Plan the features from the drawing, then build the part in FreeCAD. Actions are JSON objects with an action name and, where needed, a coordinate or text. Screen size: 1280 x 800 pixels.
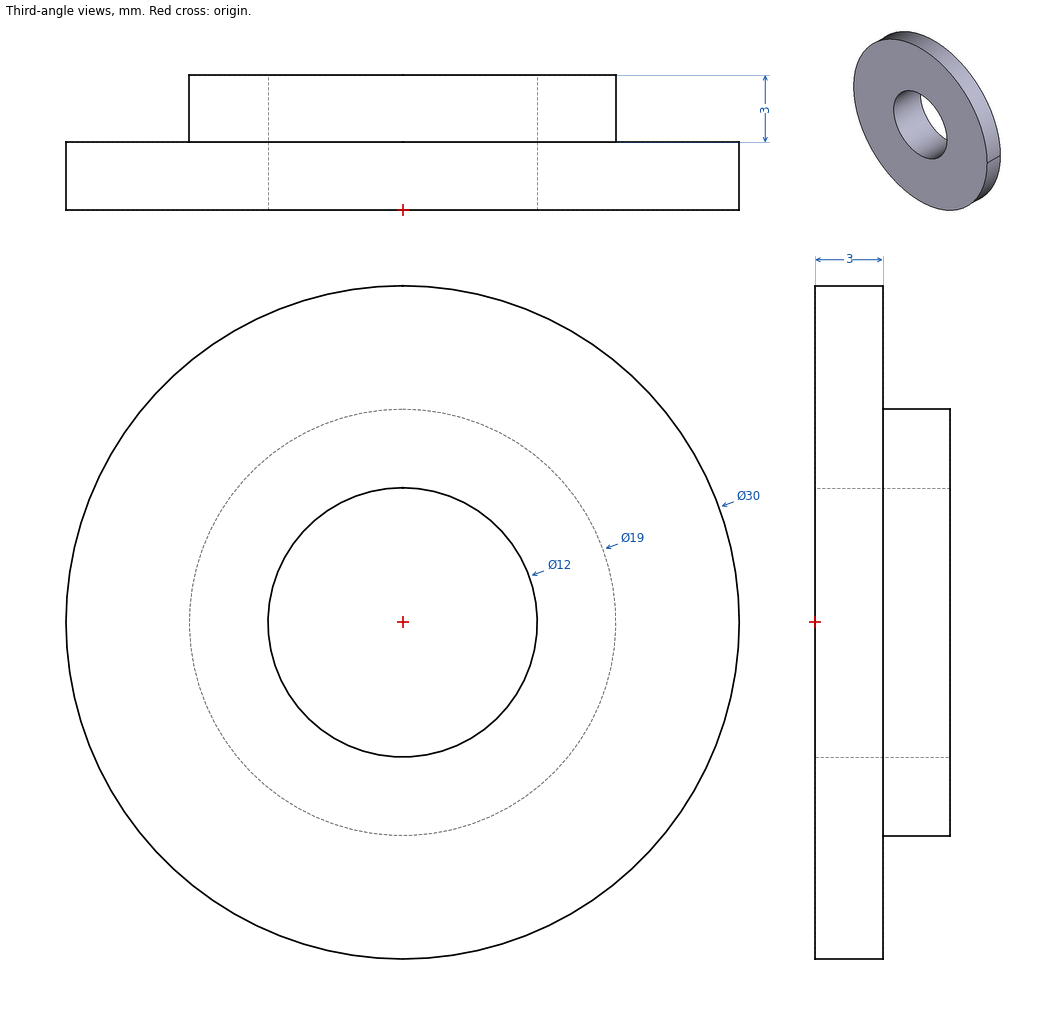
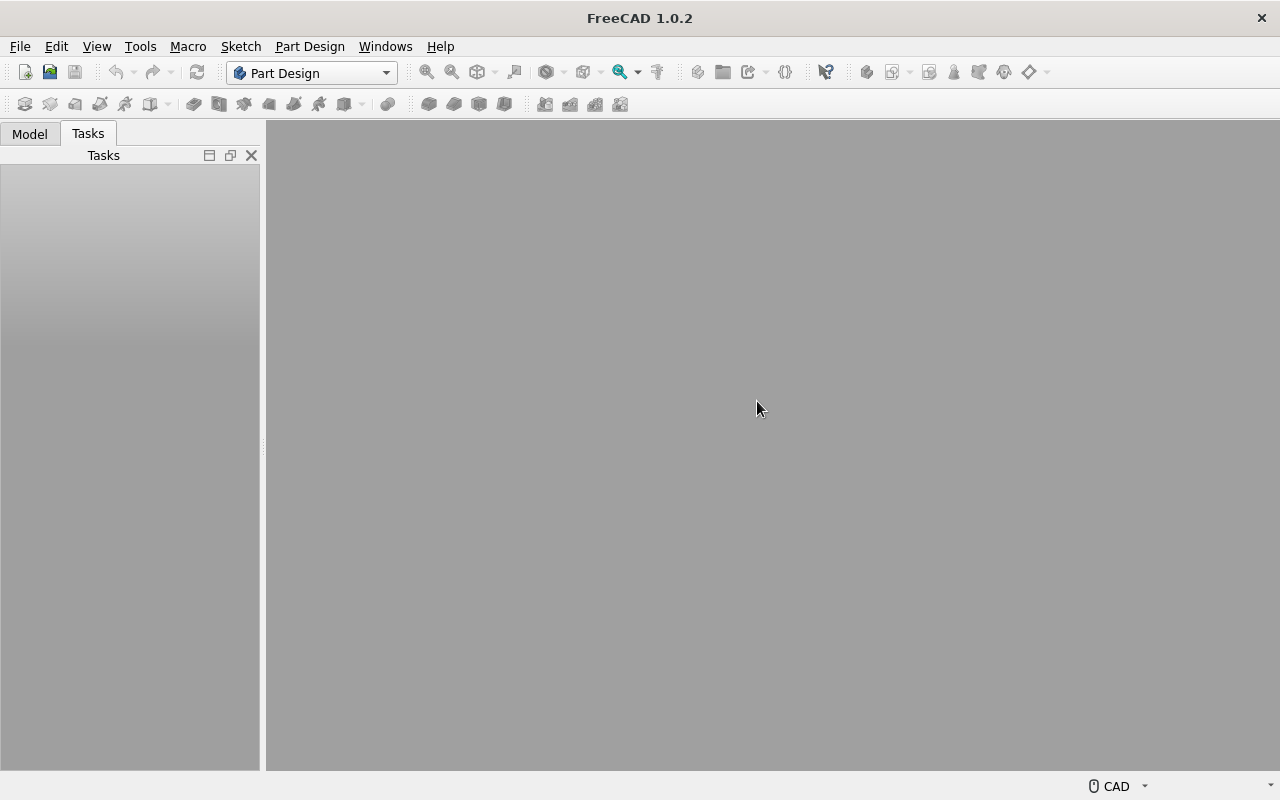
{"action": "left_click", "coordinate": [25, 72]}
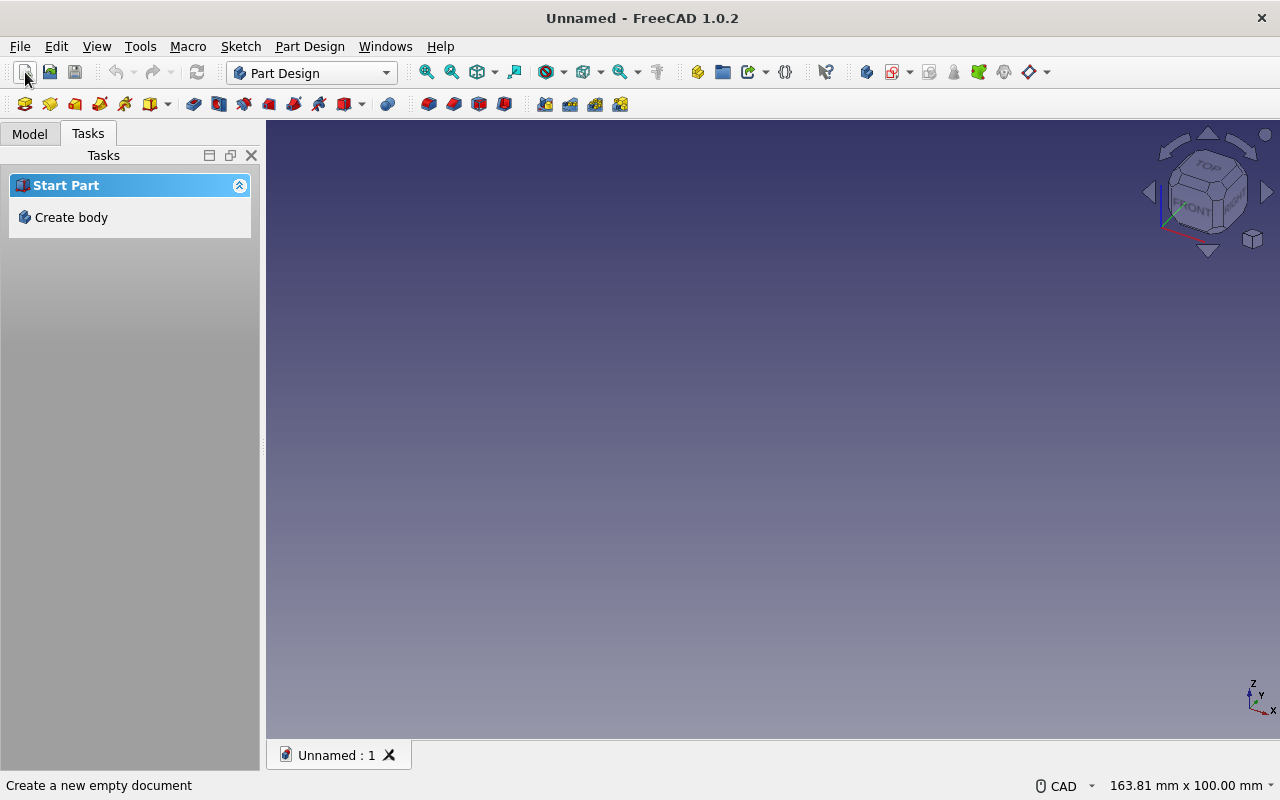
{"action": "left_click", "coordinate": [892, 72]}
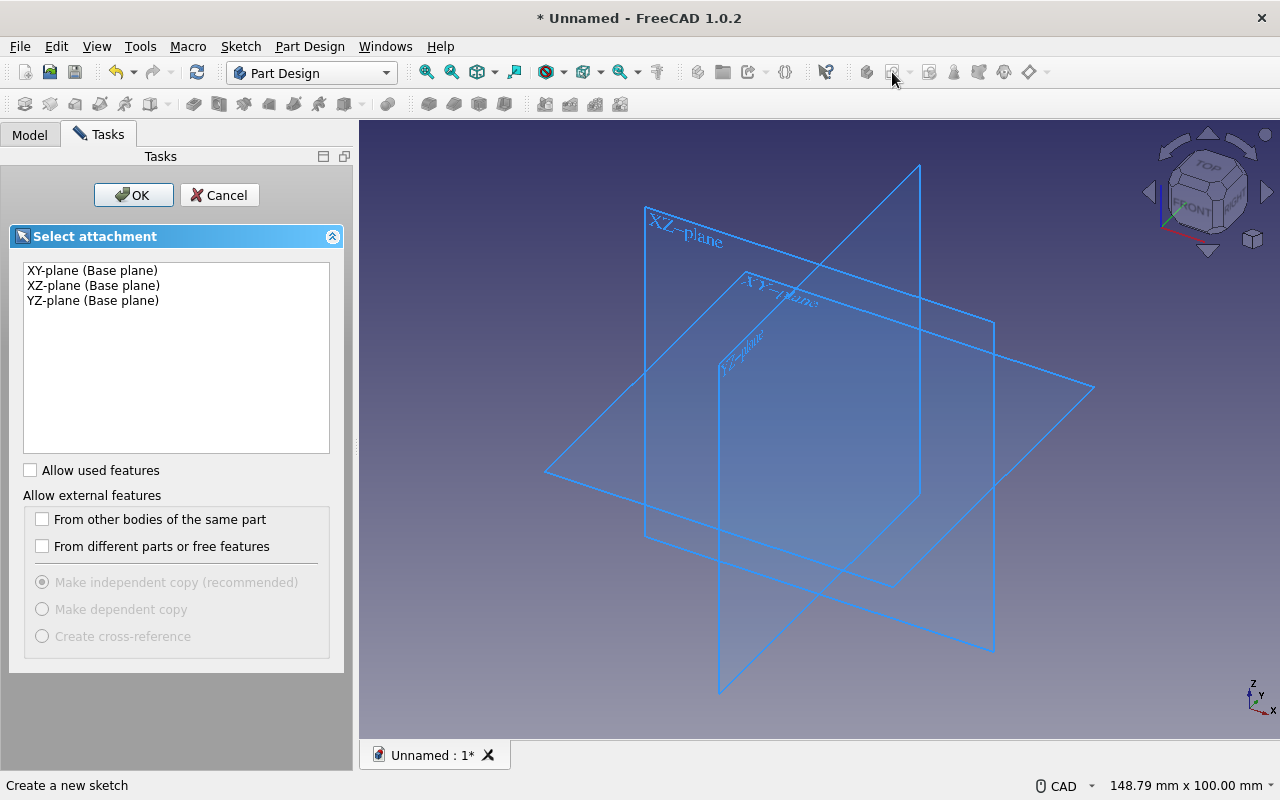
{"action": "left_click", "coordinate": [84, 286]}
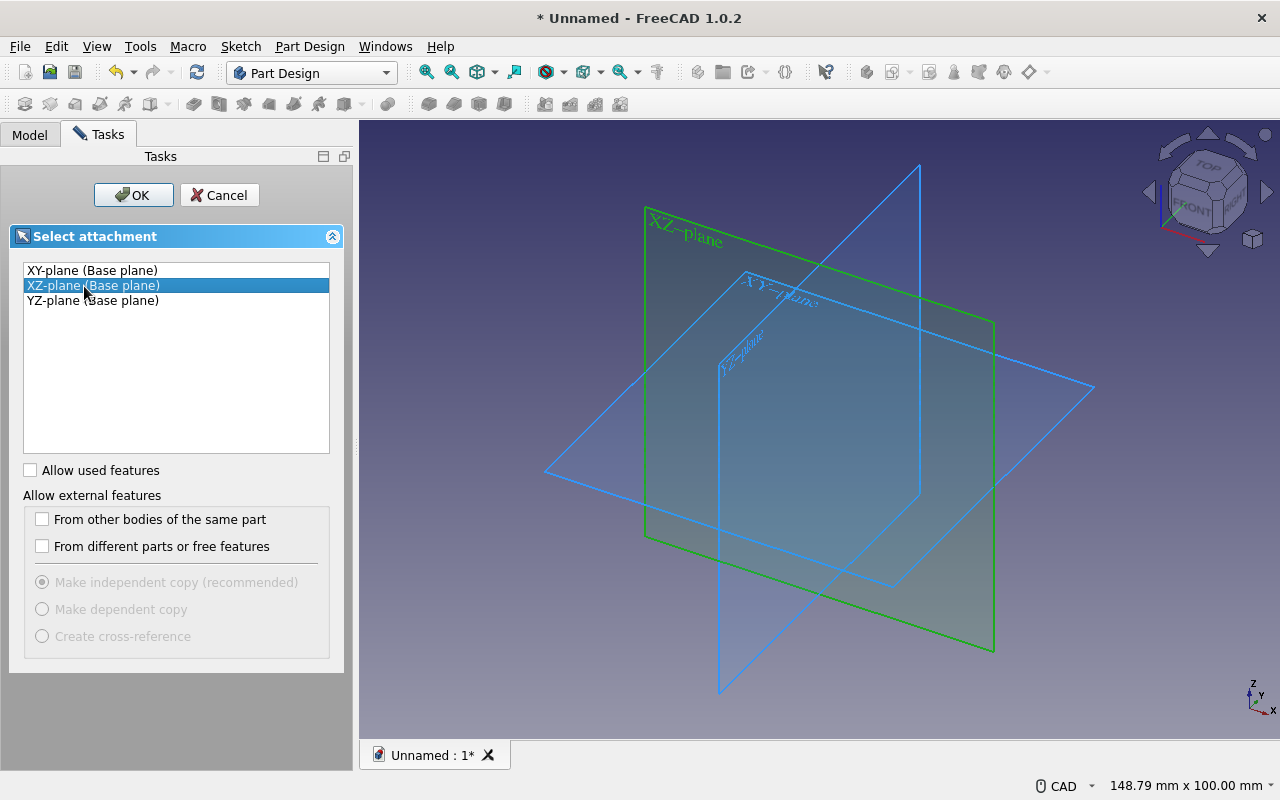
{"action": "left_click", "coordinate": [134, 195]}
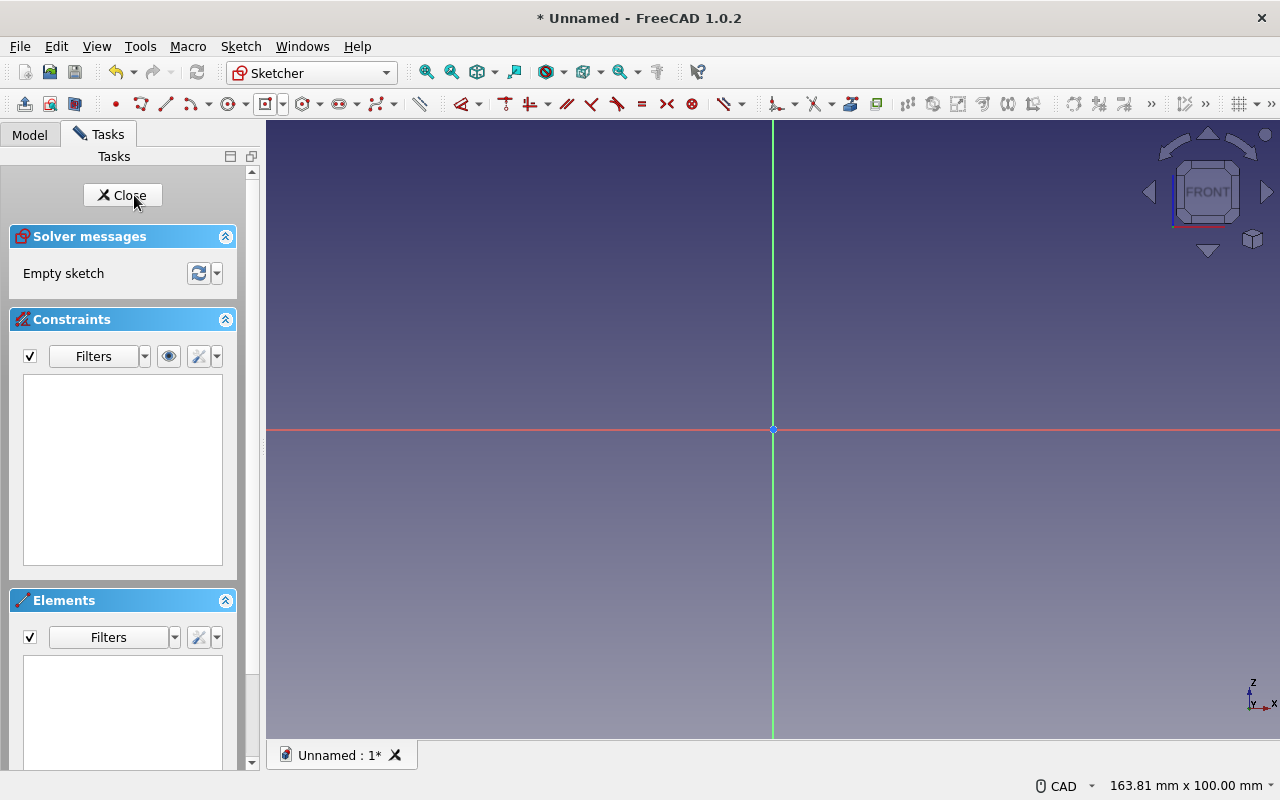
{"action": "scroll", "coordinate": [829, 430], "scroll_direction": "up", "scroll_amount": 4}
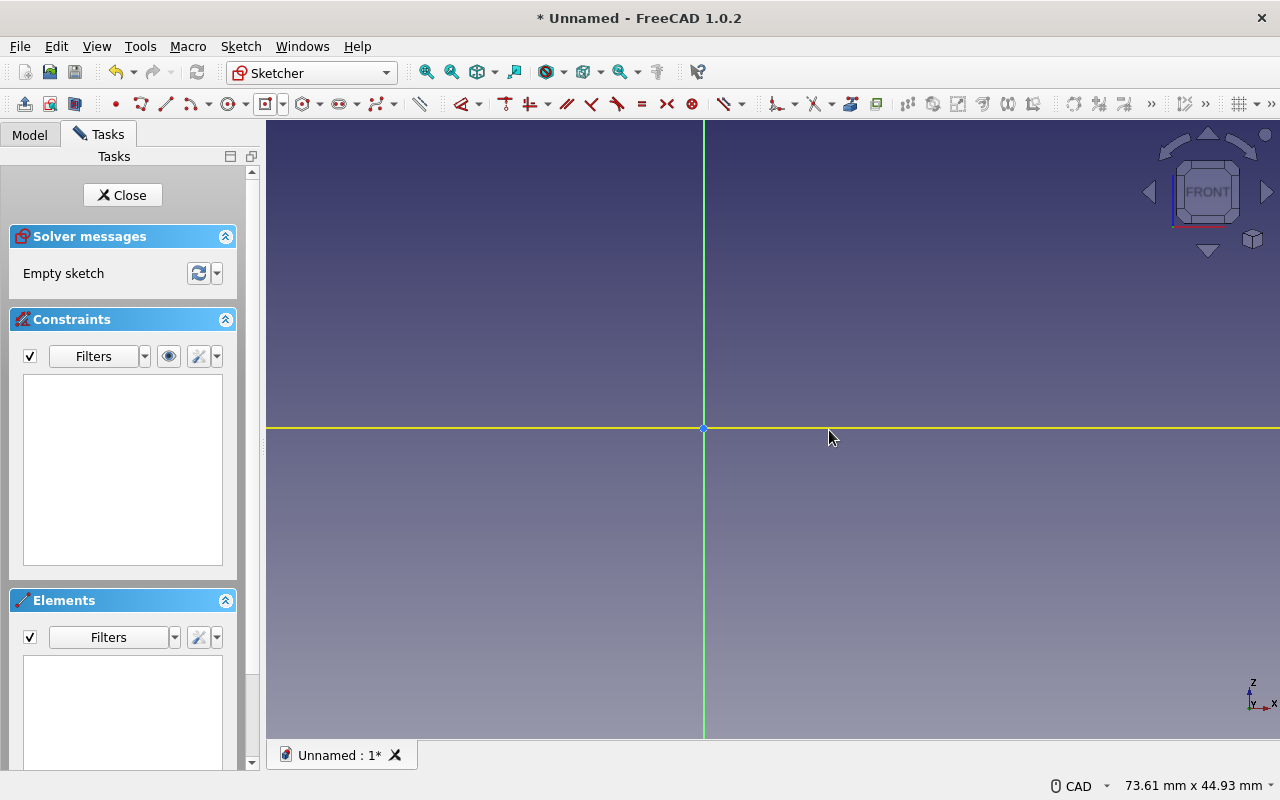
{"action": "left_click", "coordinate": [228, 104]}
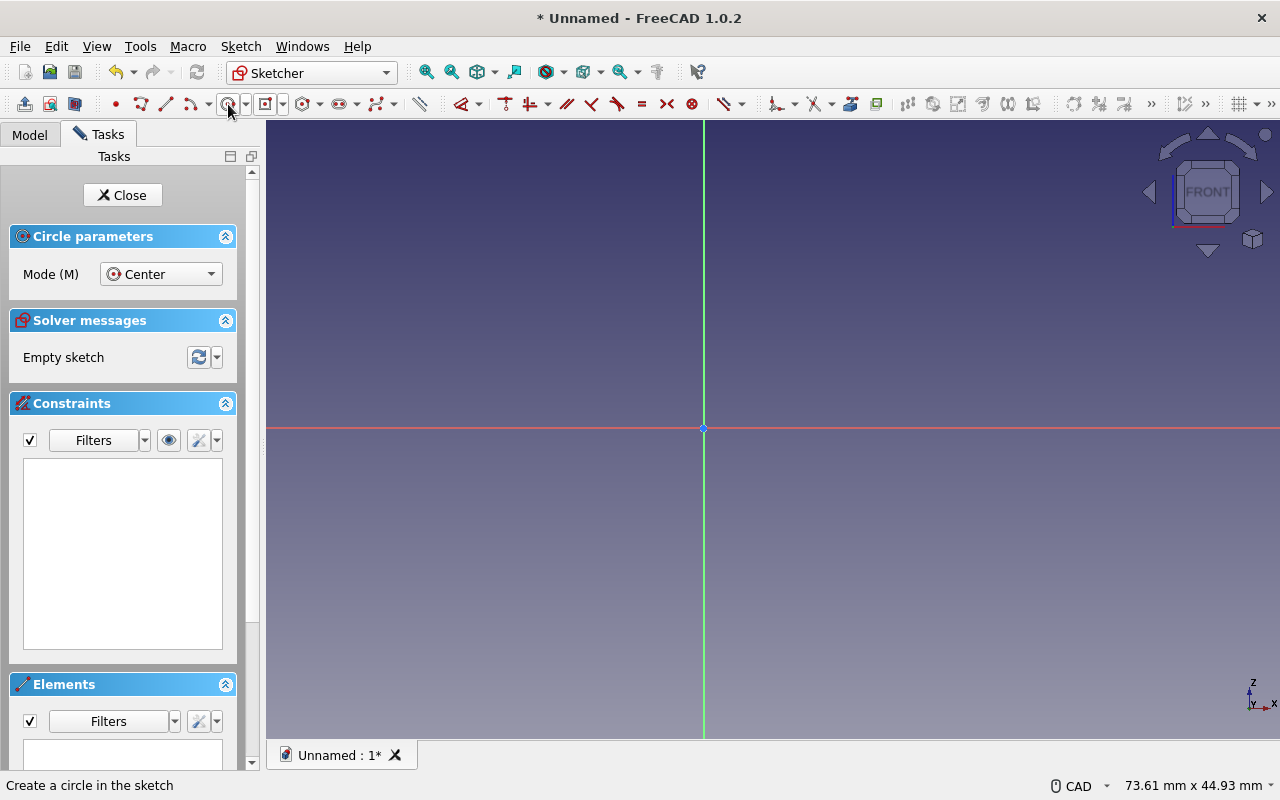
{"action": "left_click", "coordinate": [704, 428]}
{"action": "left_click", "coordinate": [850, 282]}
{"action": "key", "text": "Escape"}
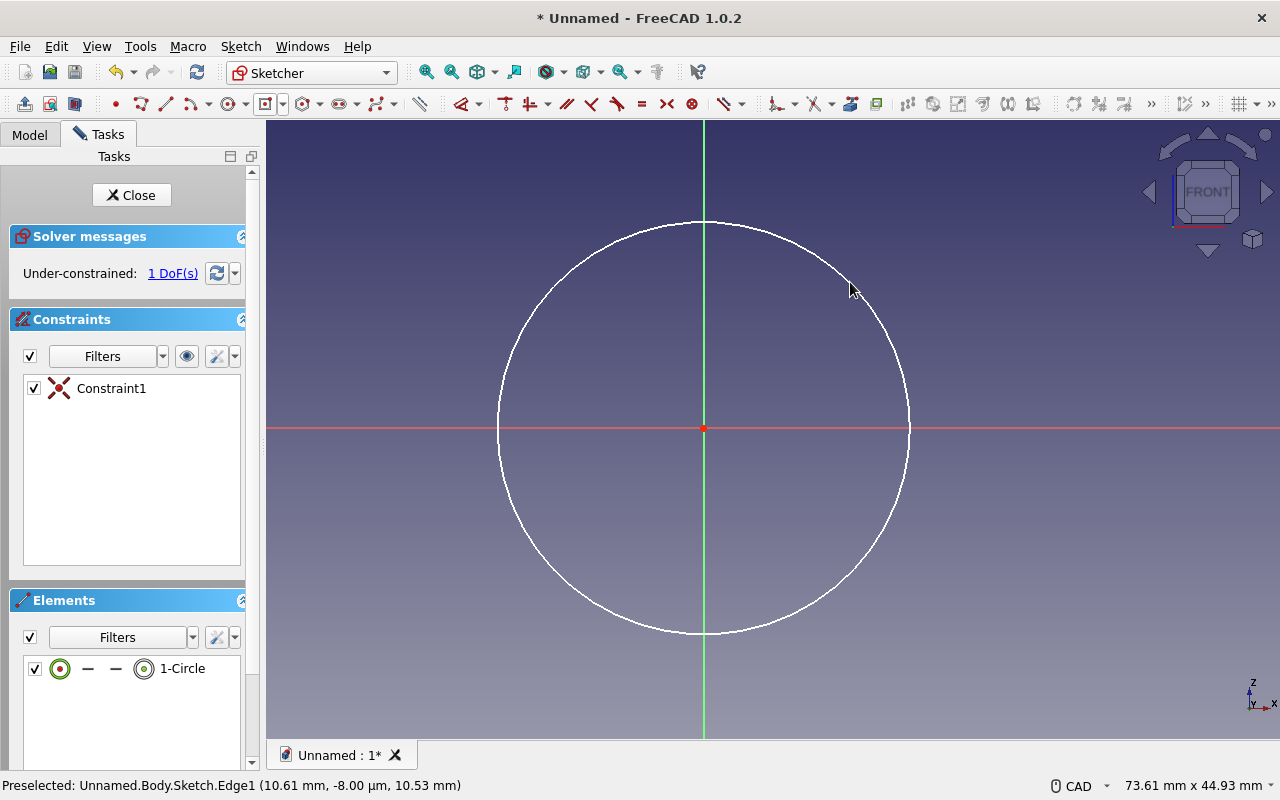
{"action": "left_click", "coordinate": [460, 104]}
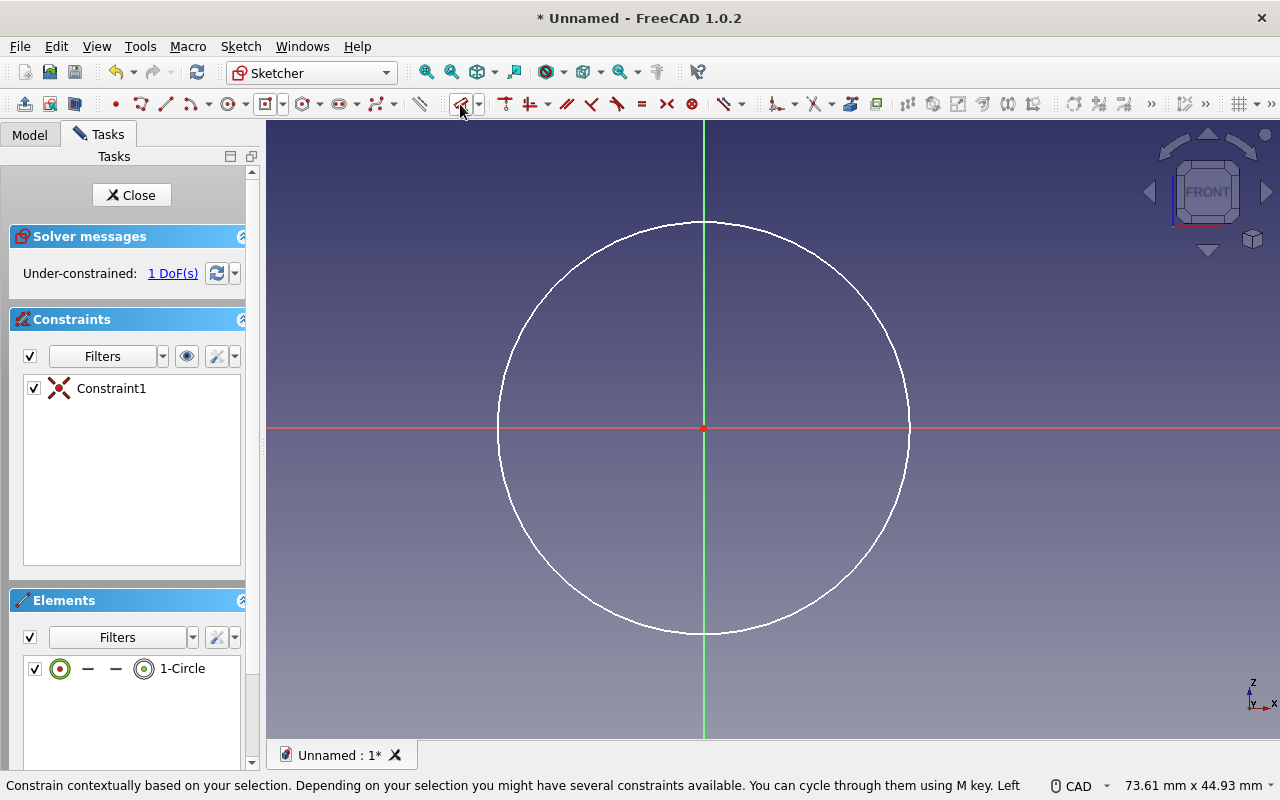
{"action": "left_click", "coordinate": [849, 282]}
{"action": "left_click", "coordinate": [872, 259]}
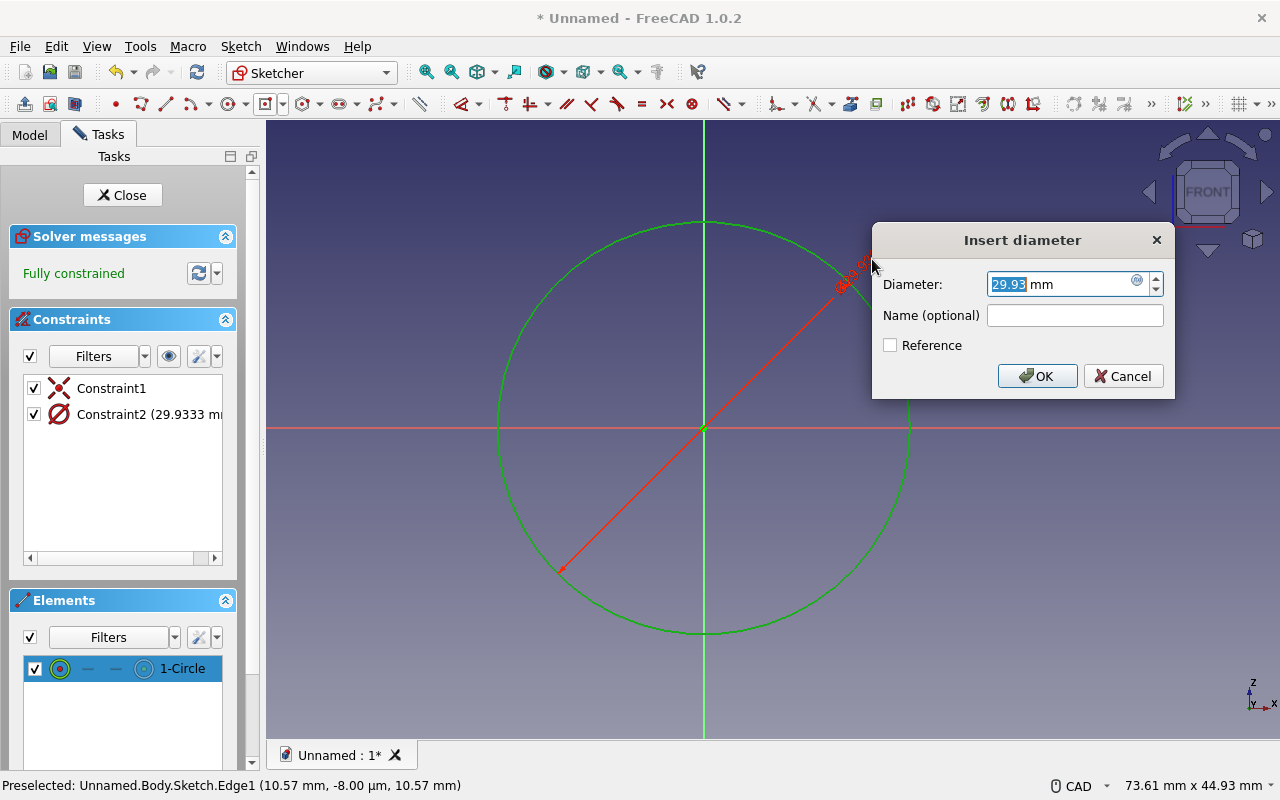
{"action": "type", "text": "30"}
{"action": "key", "text": "Return"}
{"action": "key", "text": "Escape"}